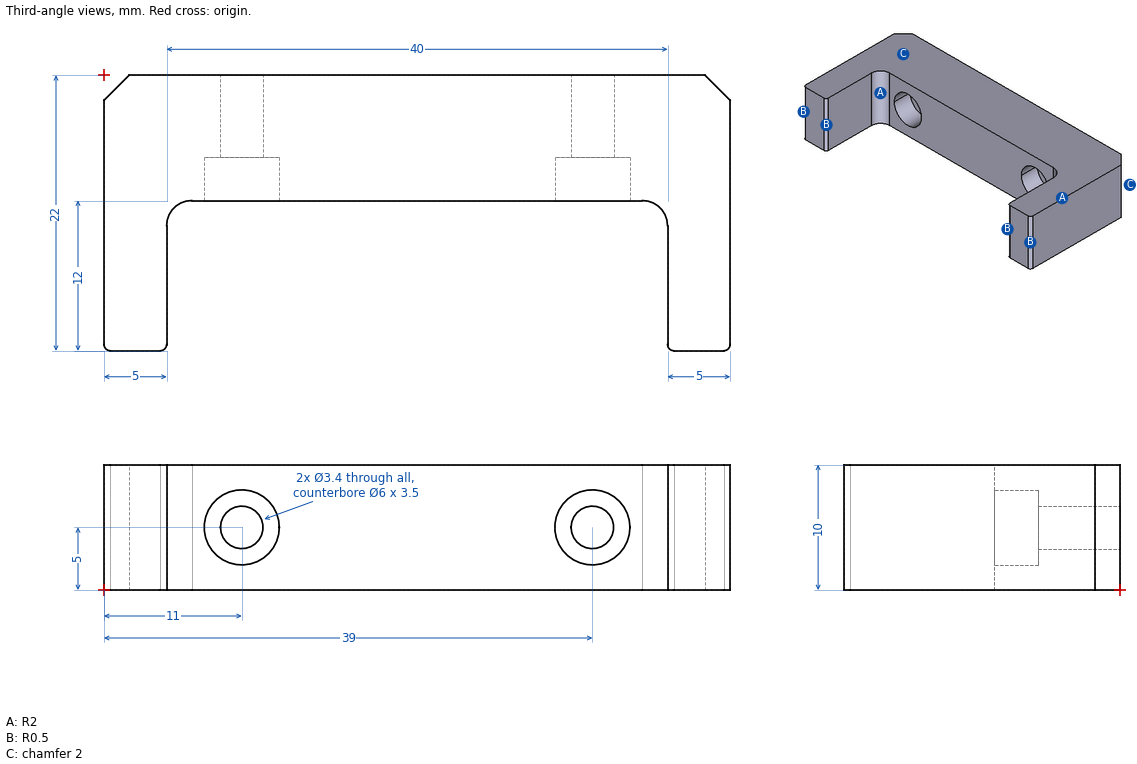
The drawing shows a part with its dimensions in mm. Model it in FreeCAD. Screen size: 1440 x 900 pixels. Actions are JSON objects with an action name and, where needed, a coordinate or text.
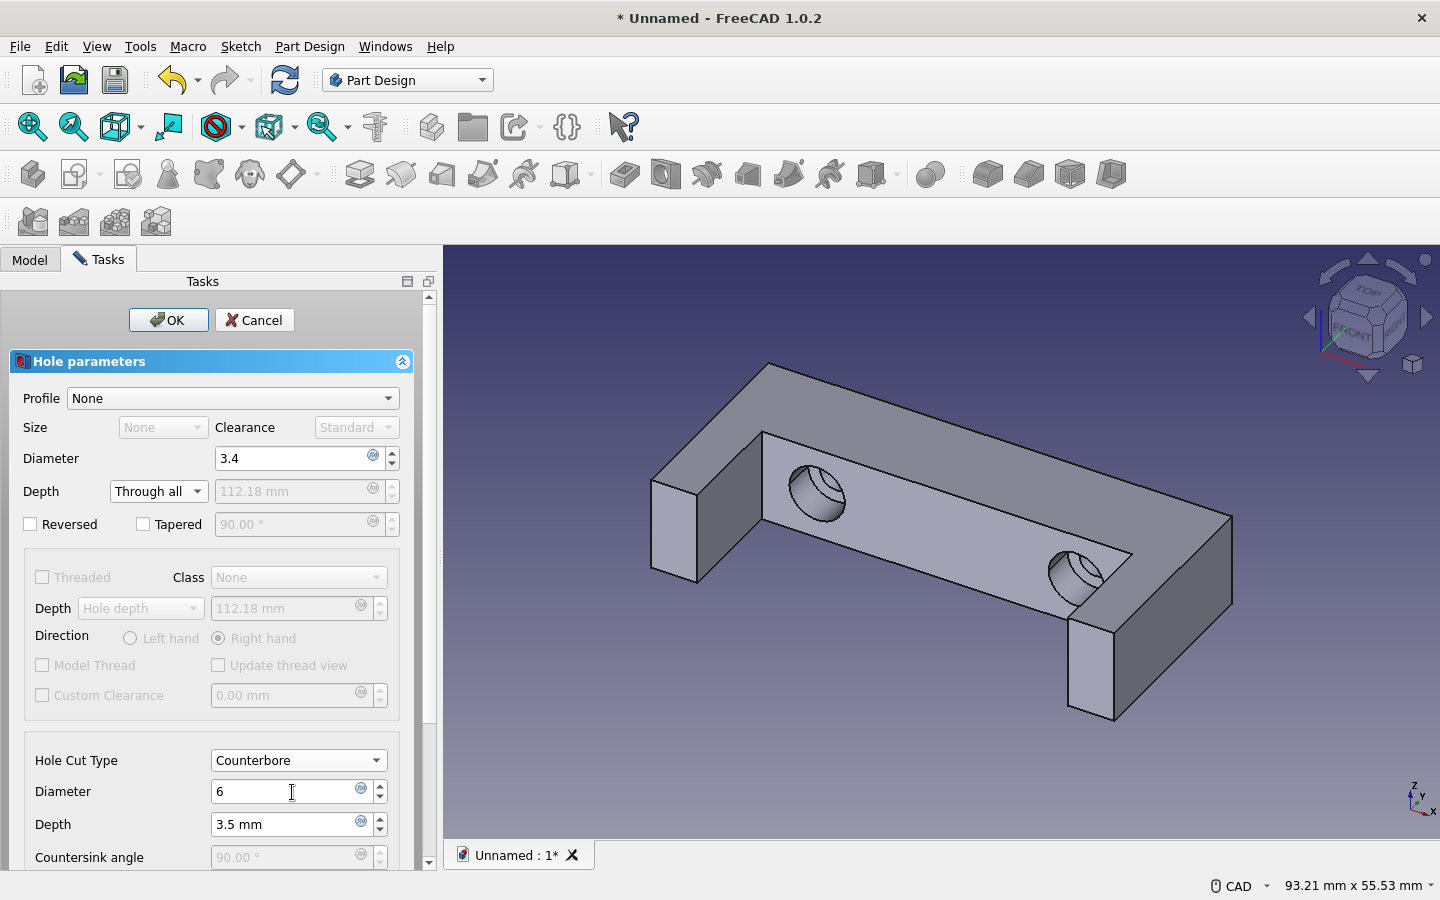
{"action": "left_click", "coordinate": [169, 320]}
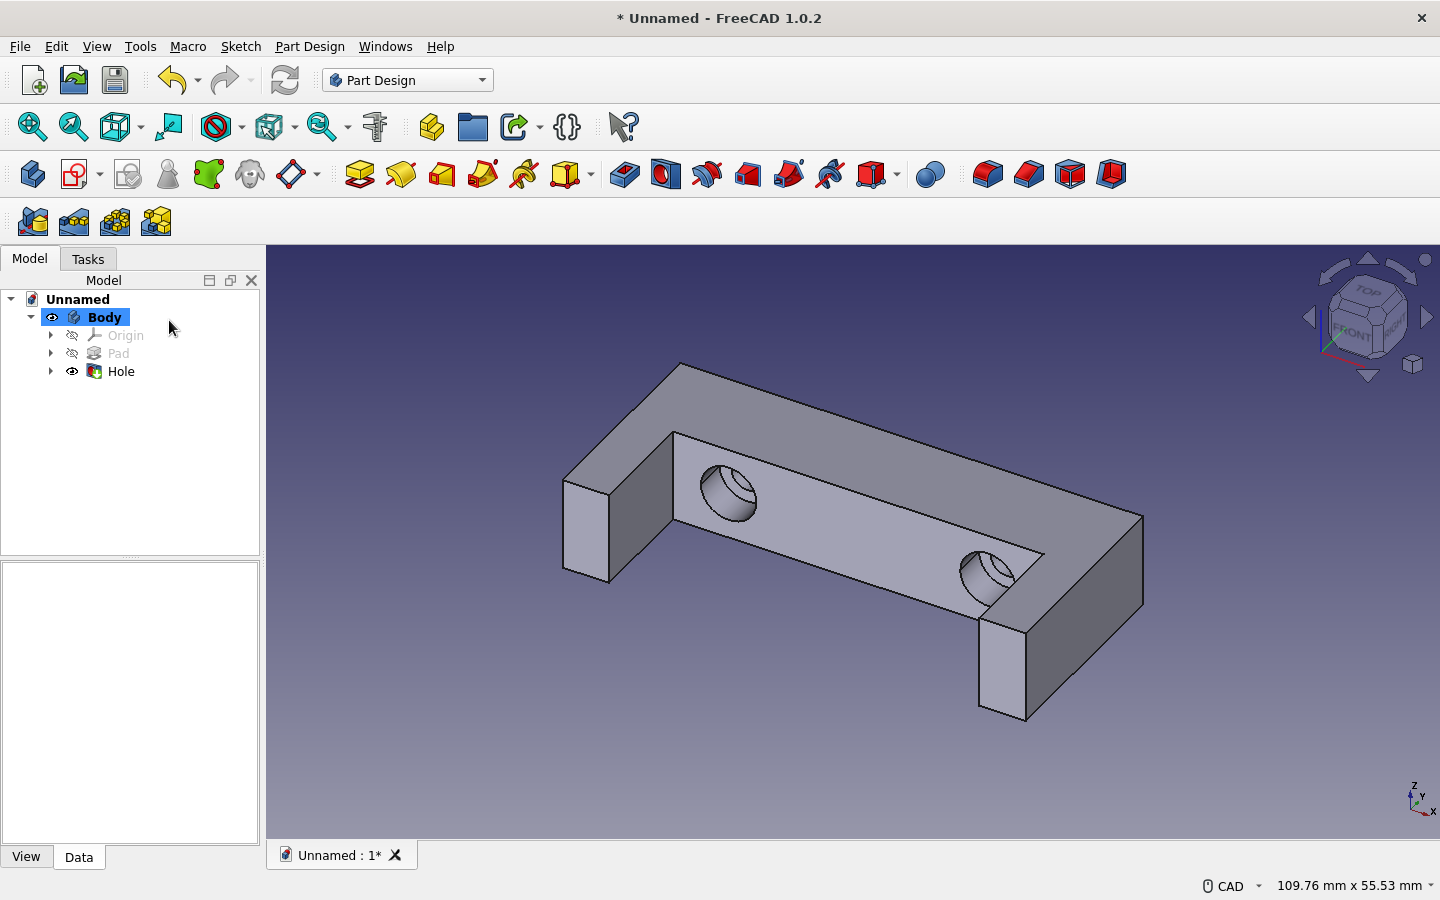
{"action": "key", "text": "0"}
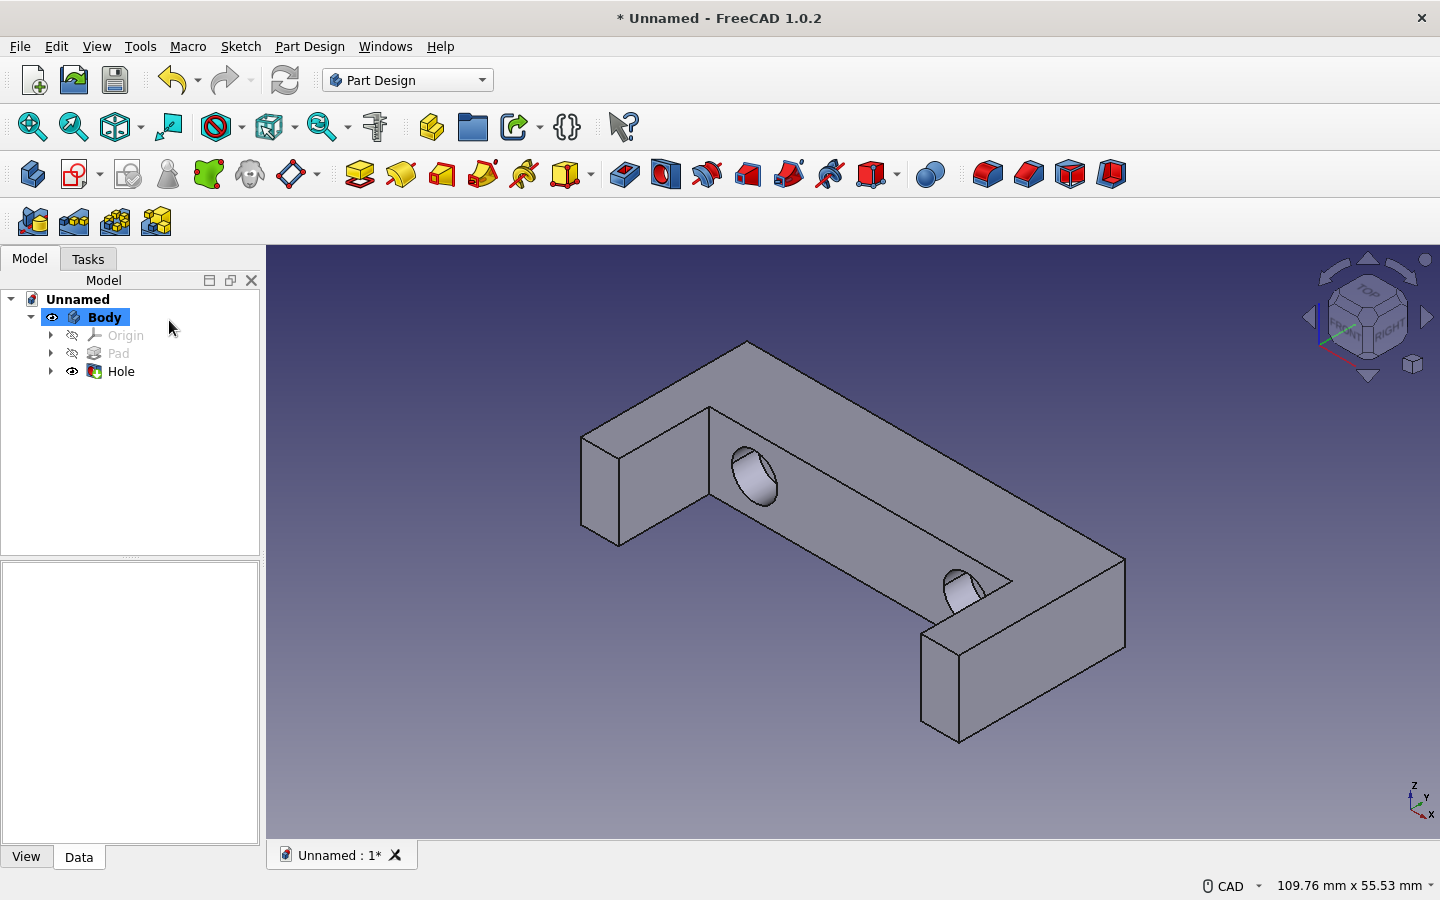
{"action": "key", "text": "2"}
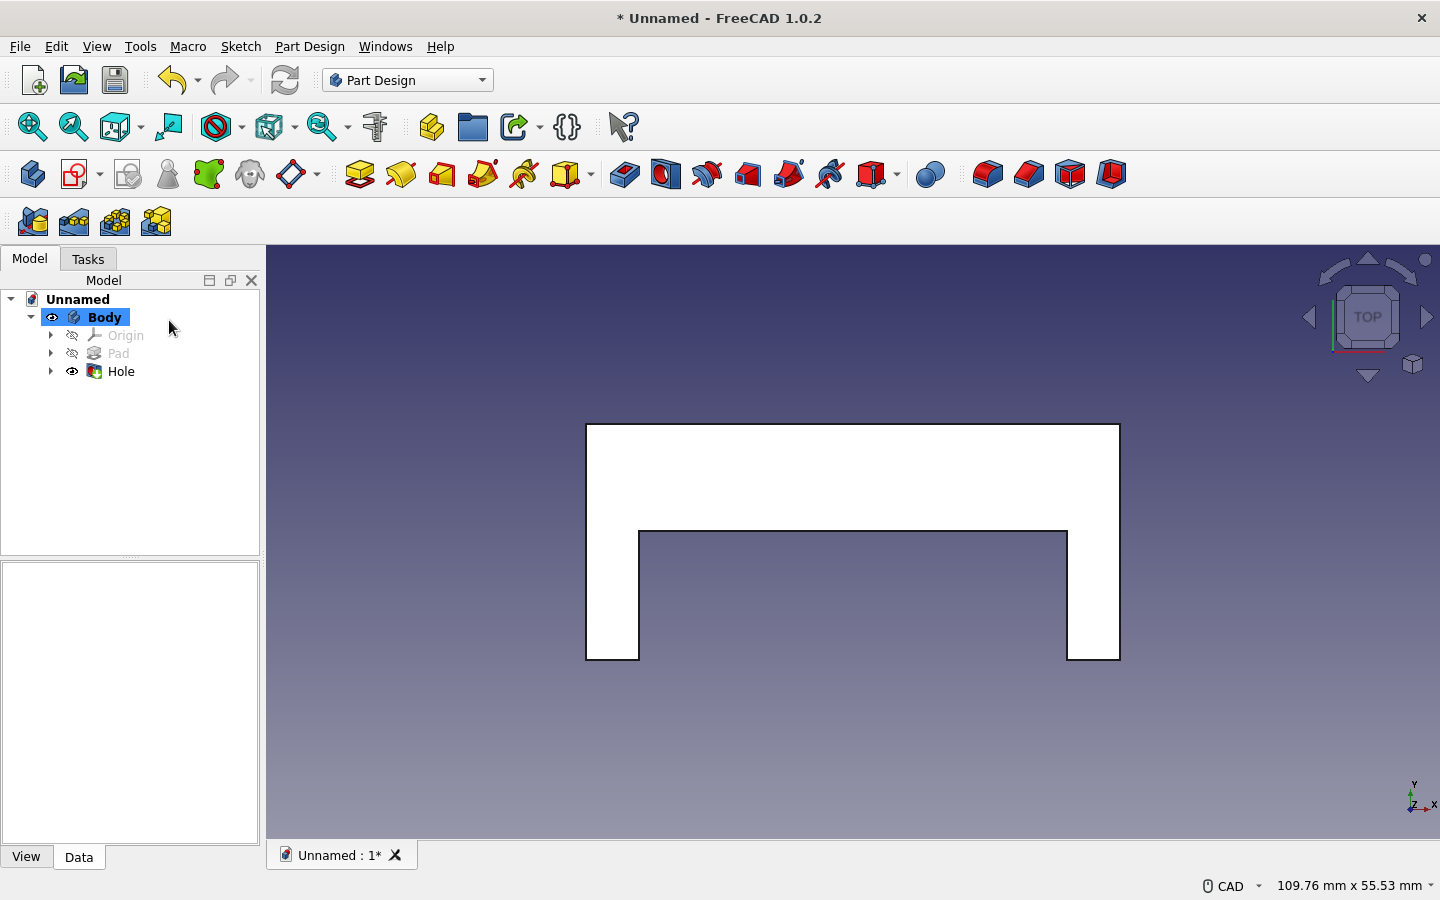
{"action": "key", "text": "1"}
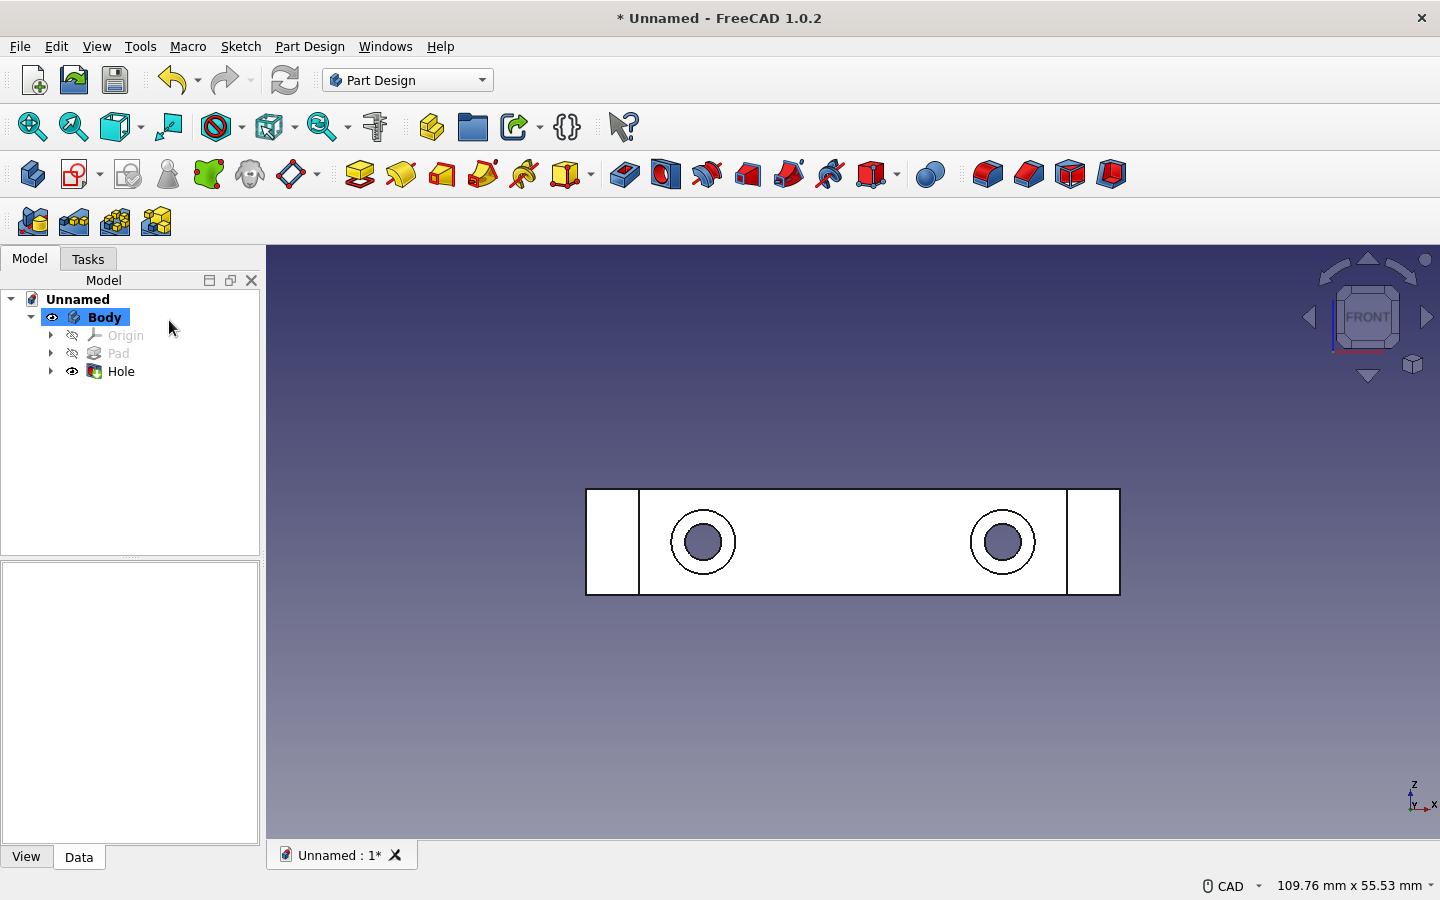
{"action": "key", "text": "3"}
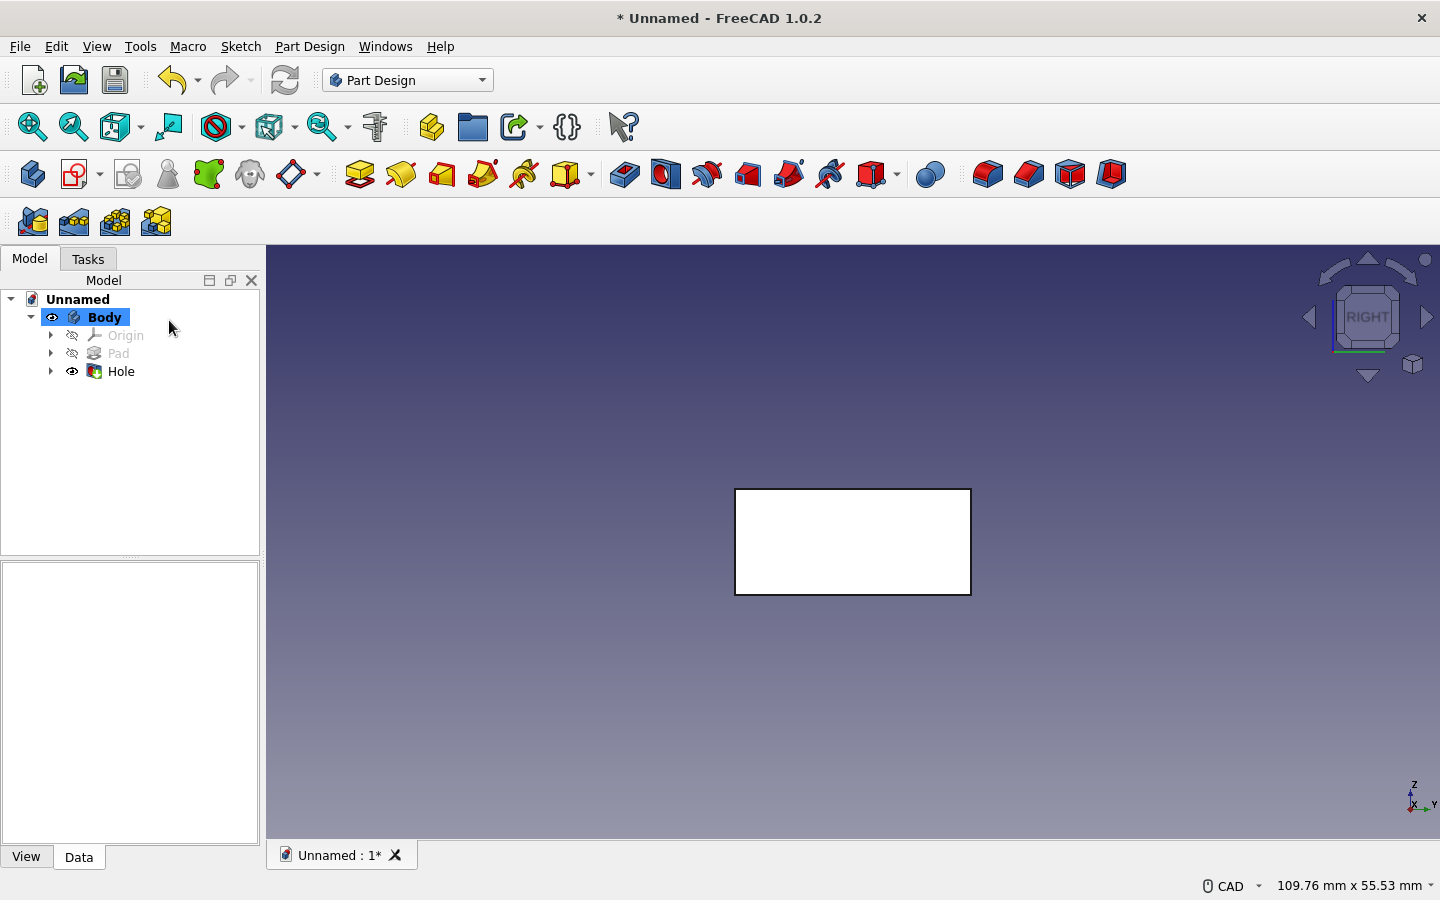
{"action": "left_click", "coordinate": [33, 128]}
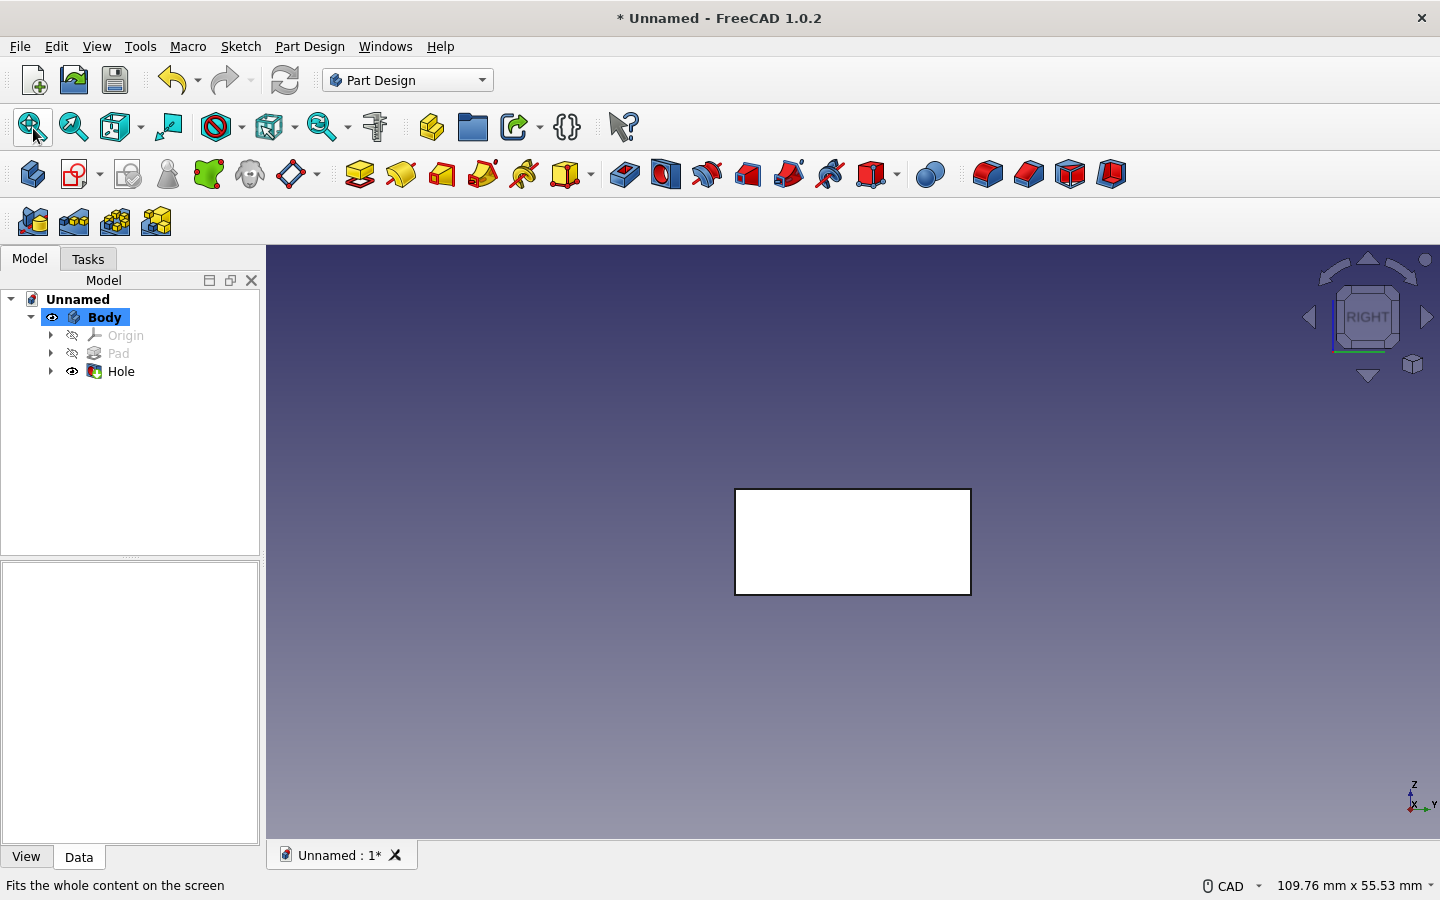
{"action": "key", "text": "5"}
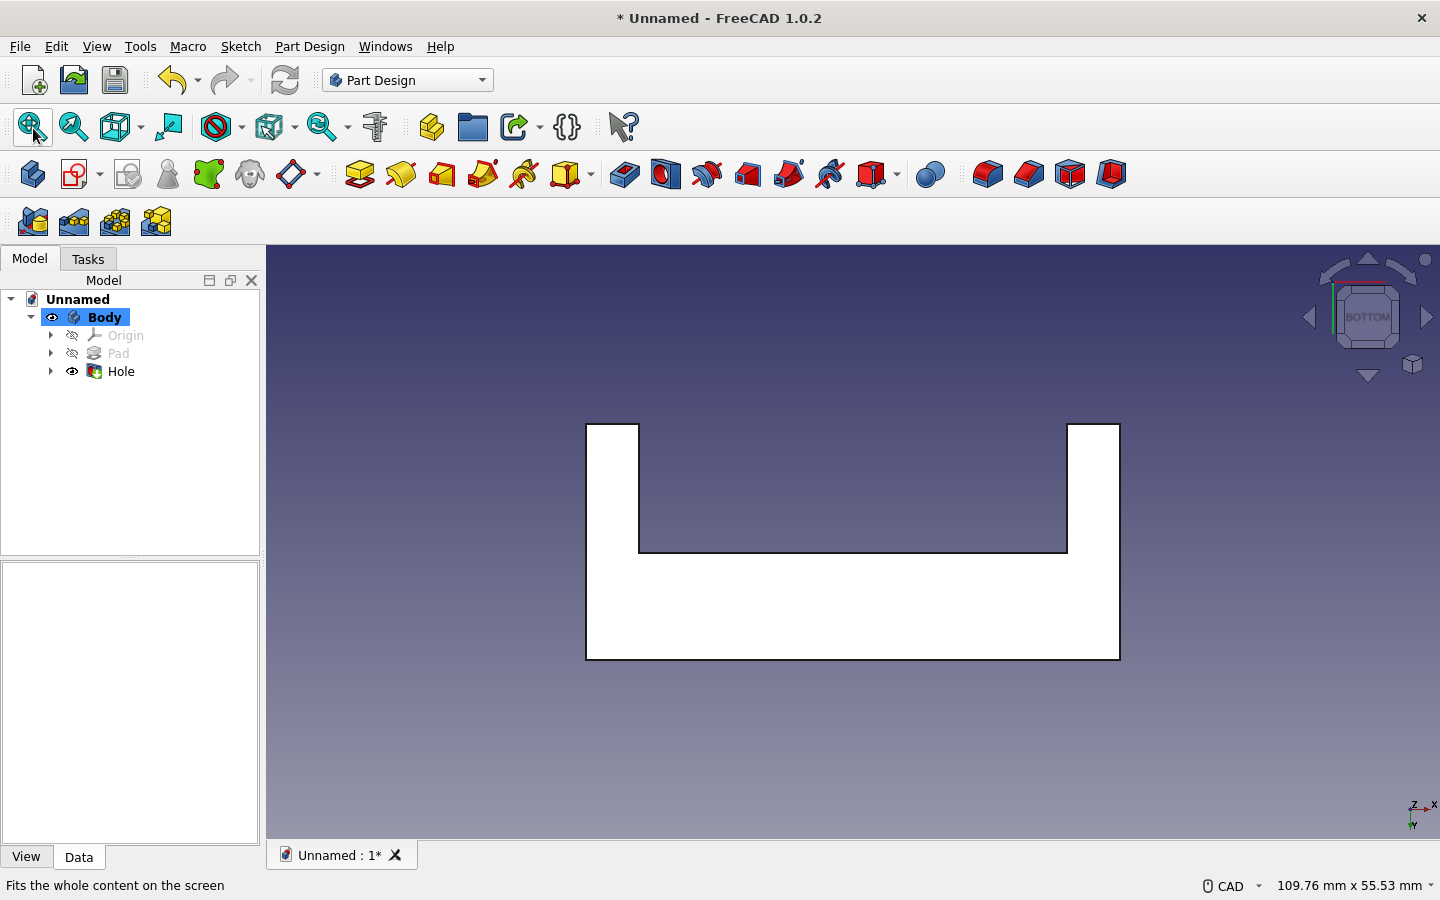
{"action": "key", "text": "4"}